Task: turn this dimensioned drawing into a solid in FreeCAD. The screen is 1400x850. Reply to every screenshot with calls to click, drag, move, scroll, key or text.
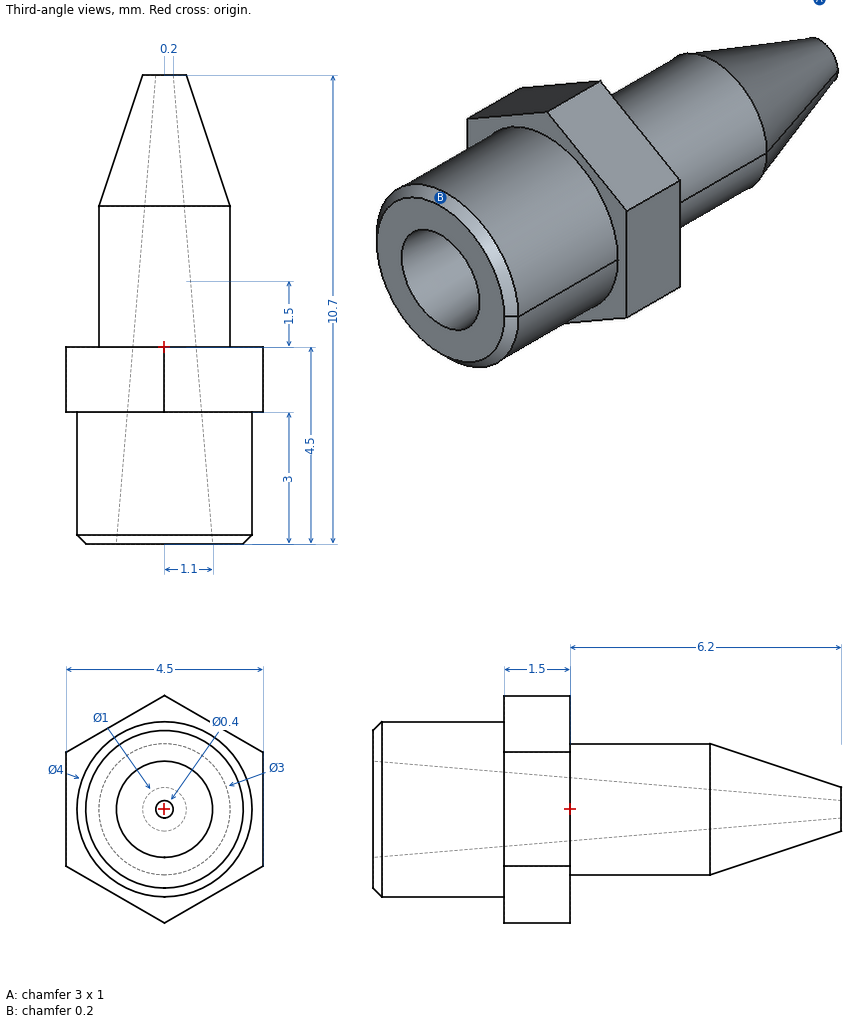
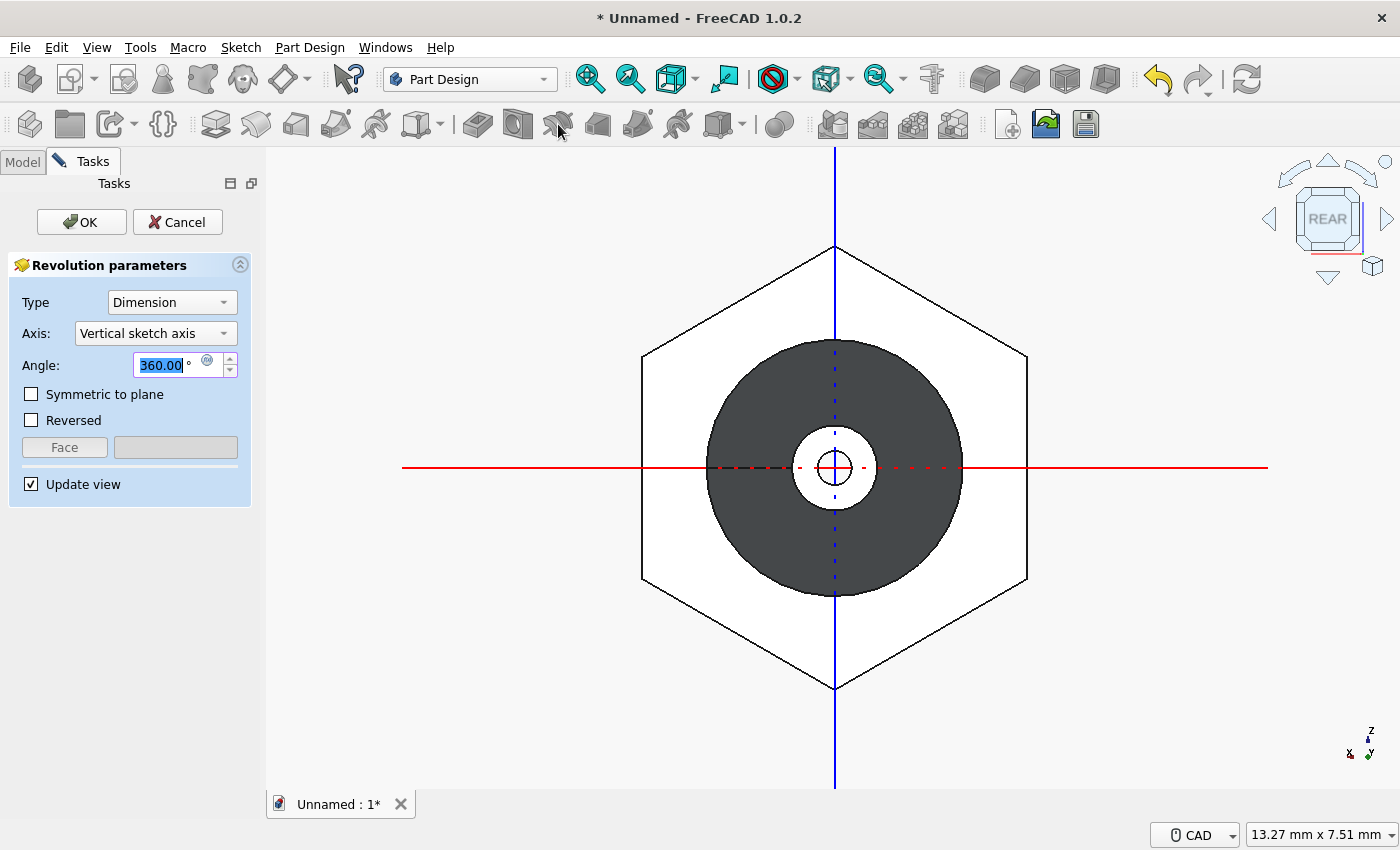
click(82, 222)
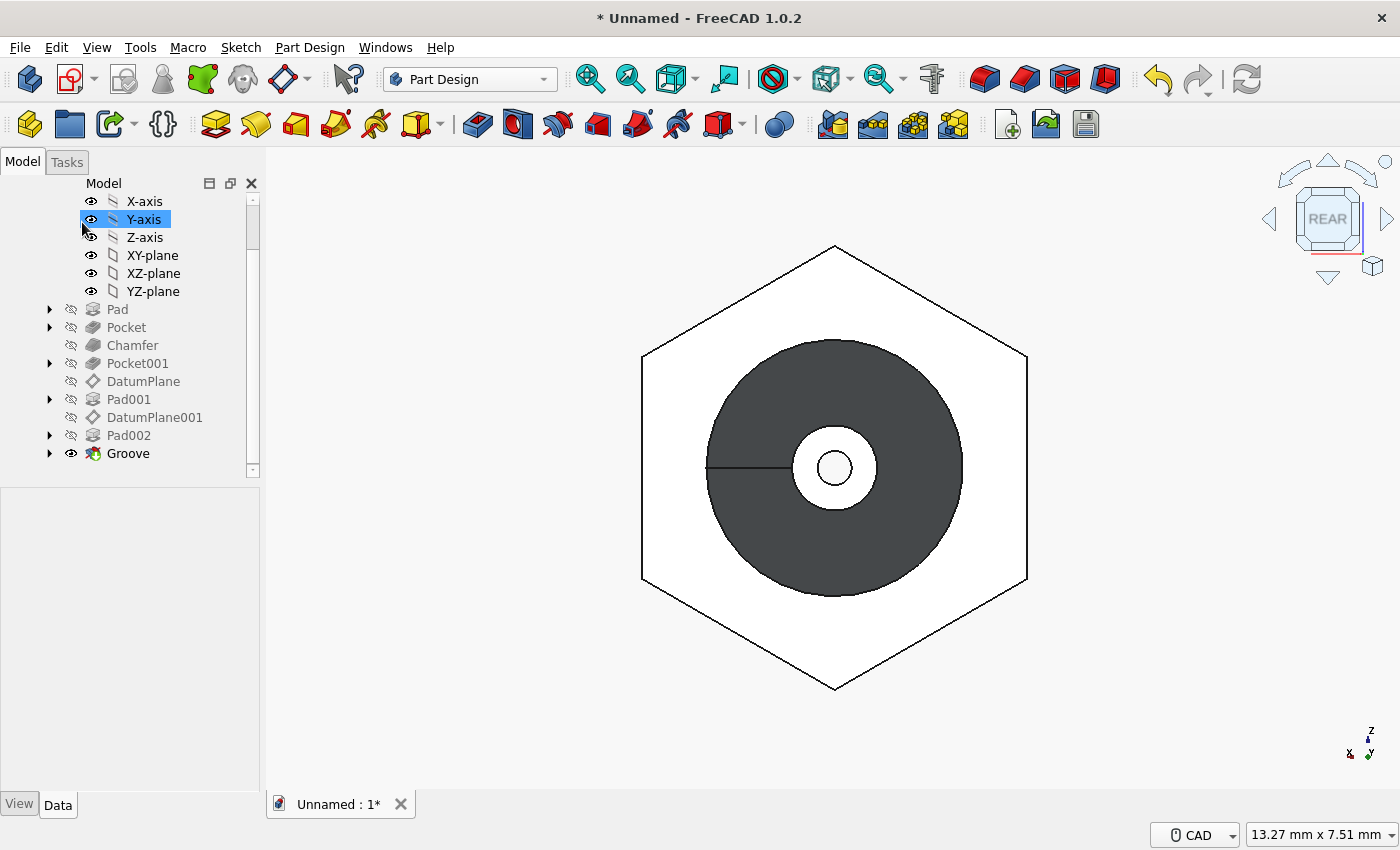
key(0)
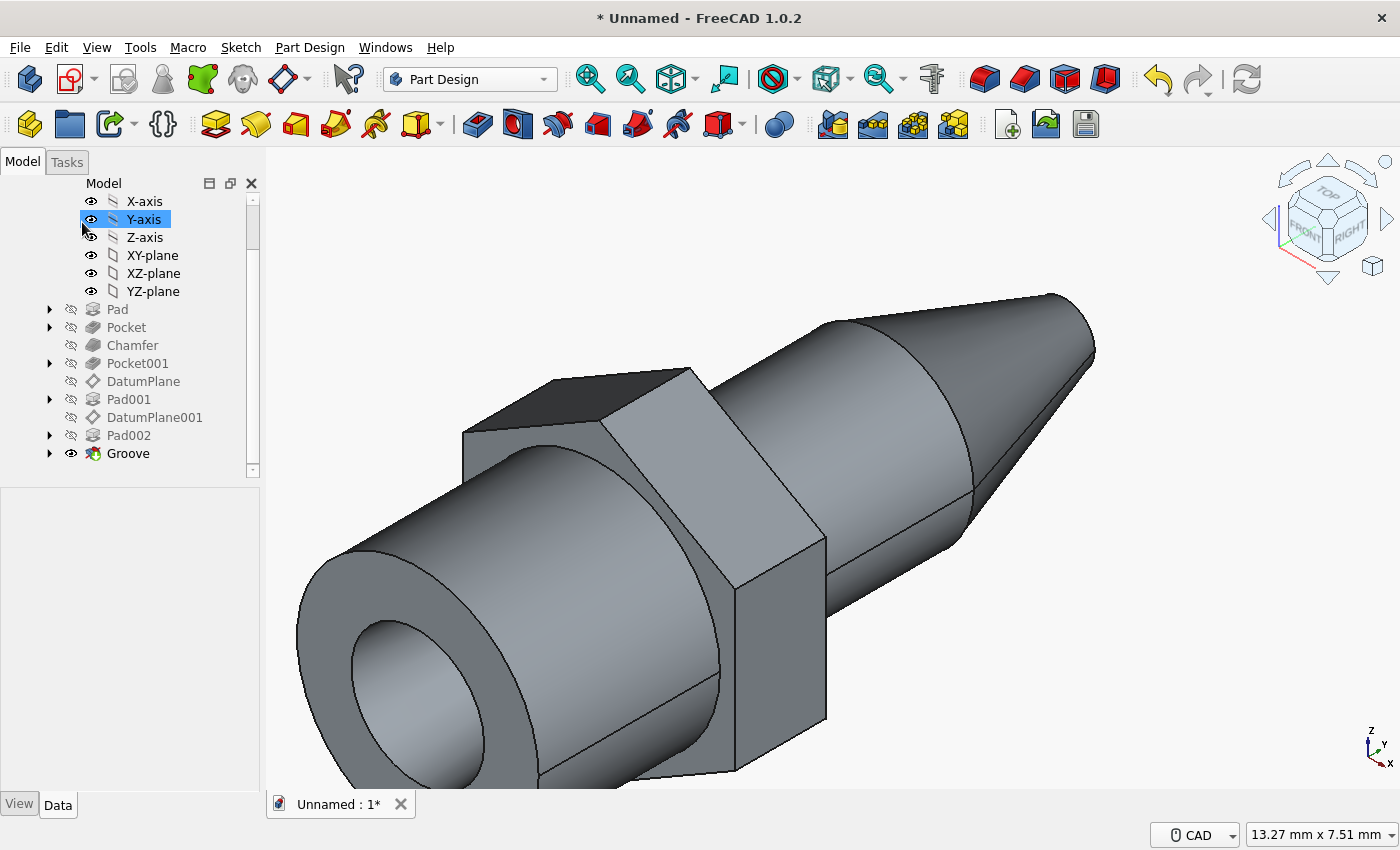
click(592, 80)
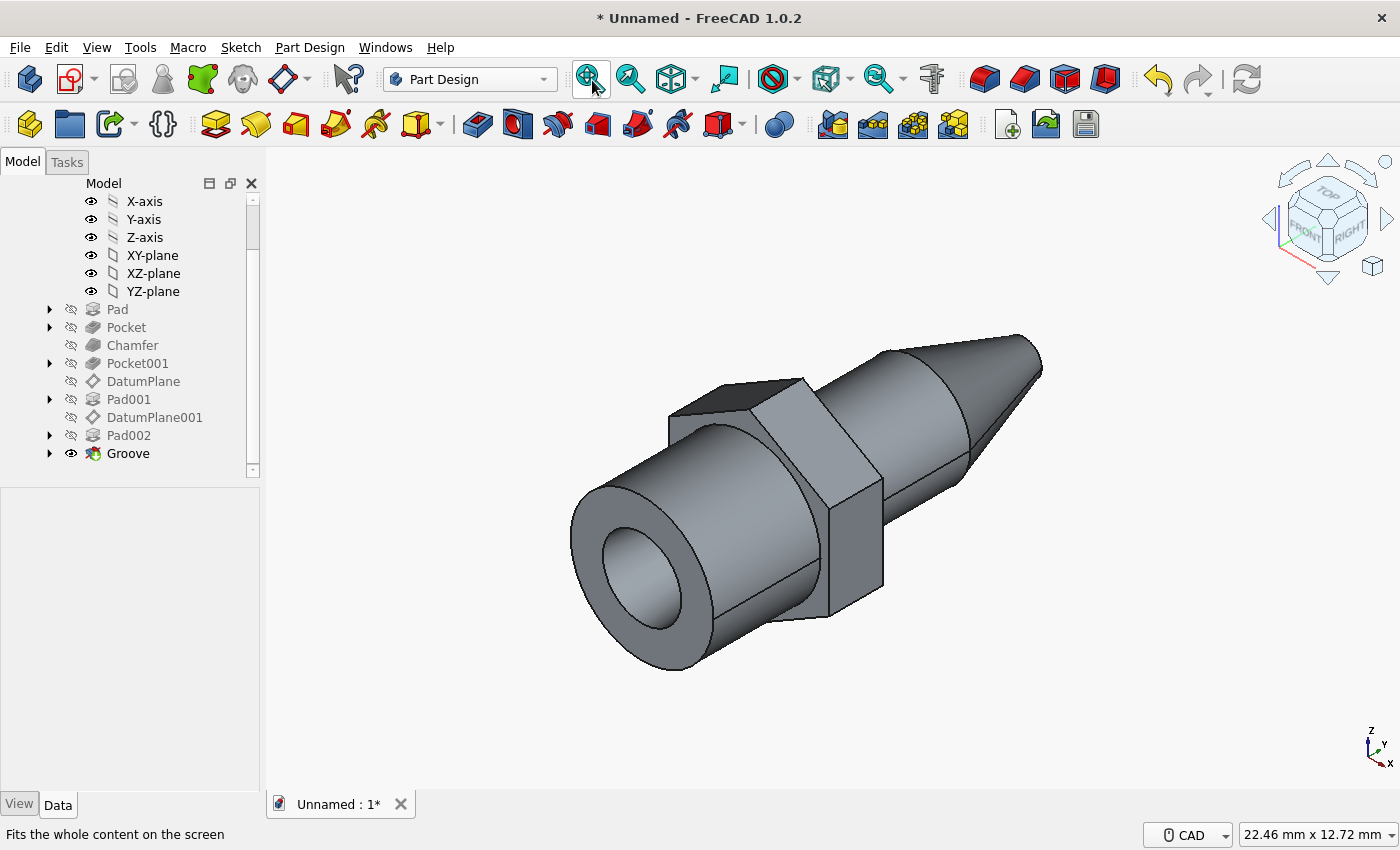
click(620, 486)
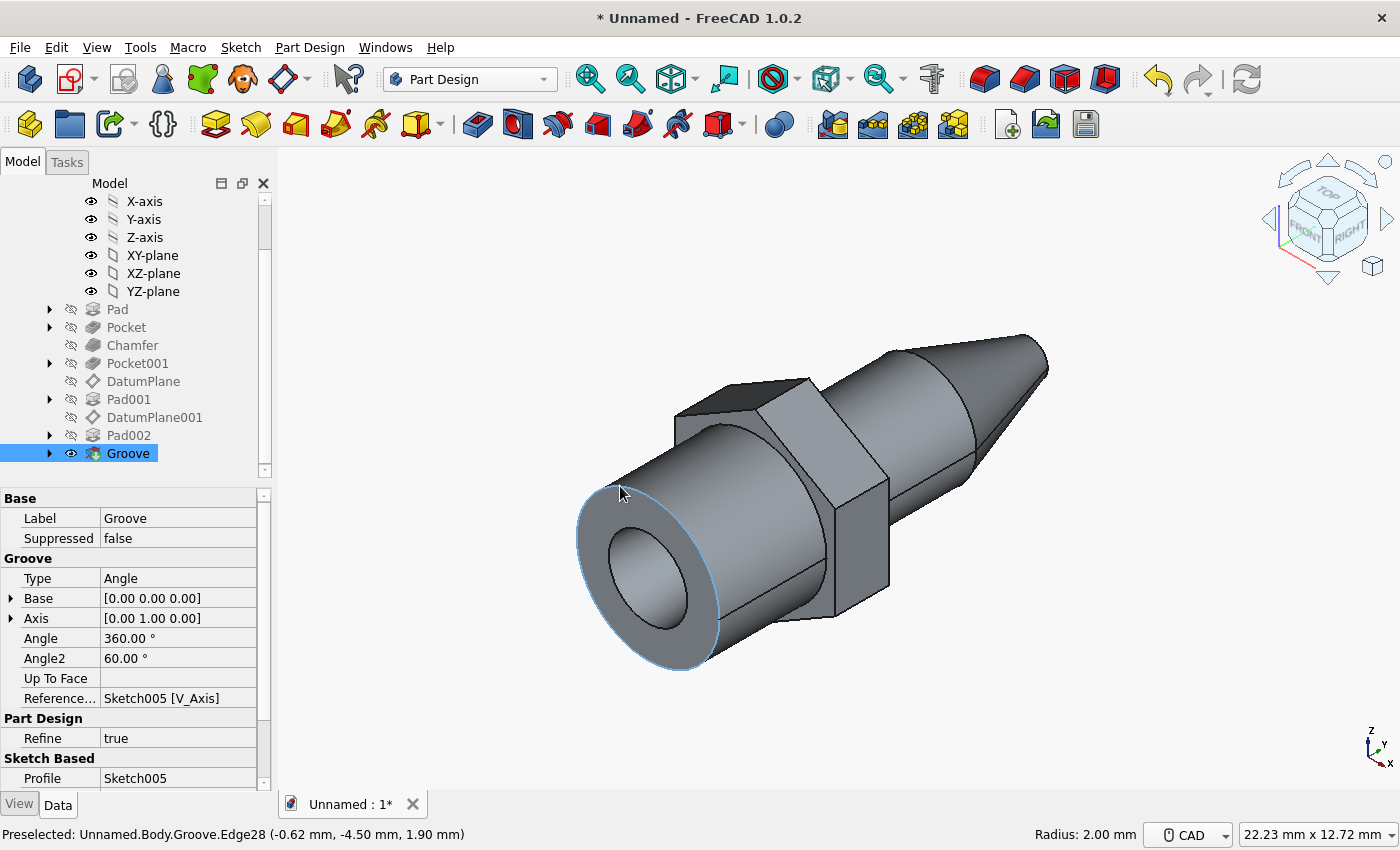
click(1026, 80)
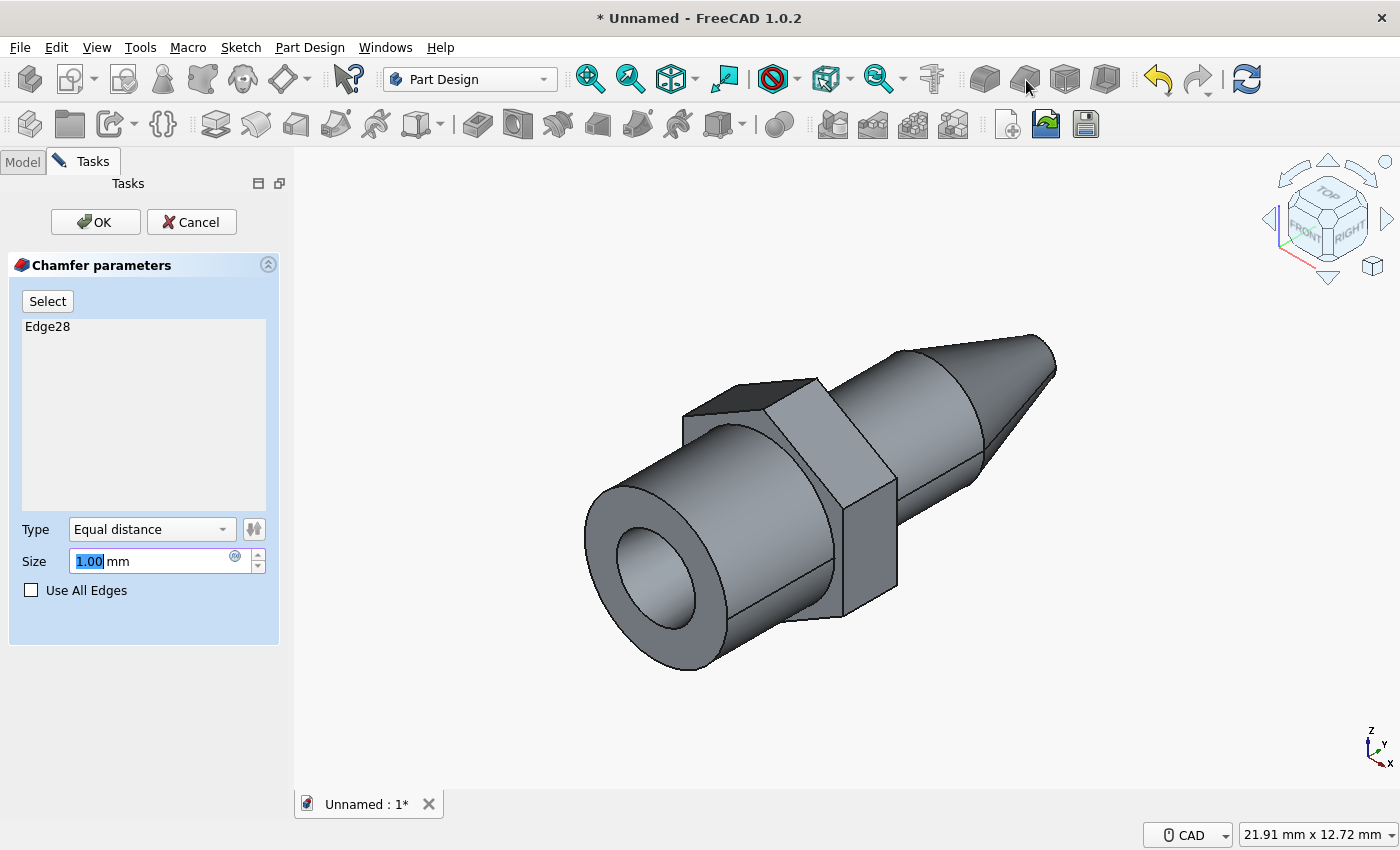
text(0.2)
key(Tab)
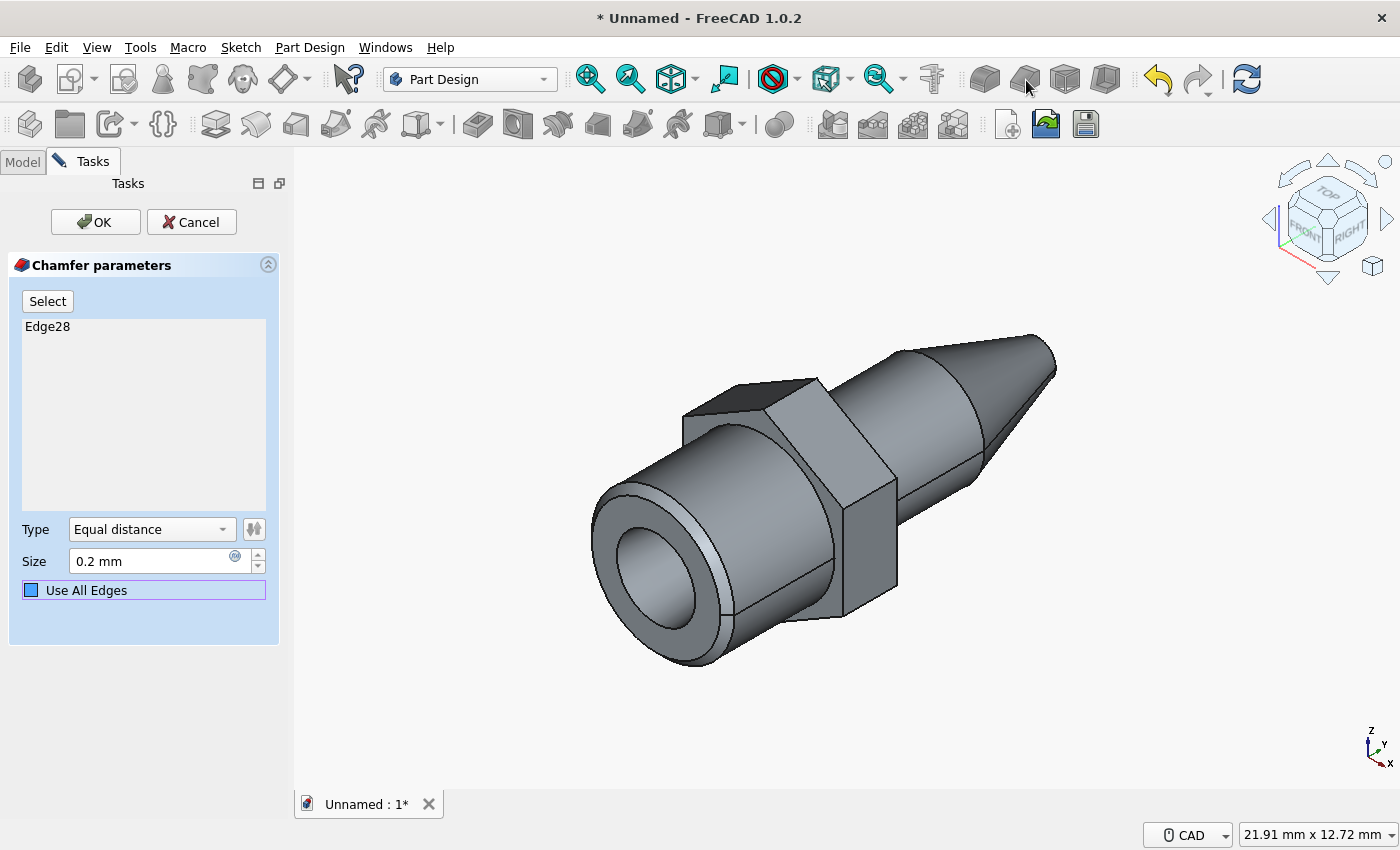
click(96, 222)